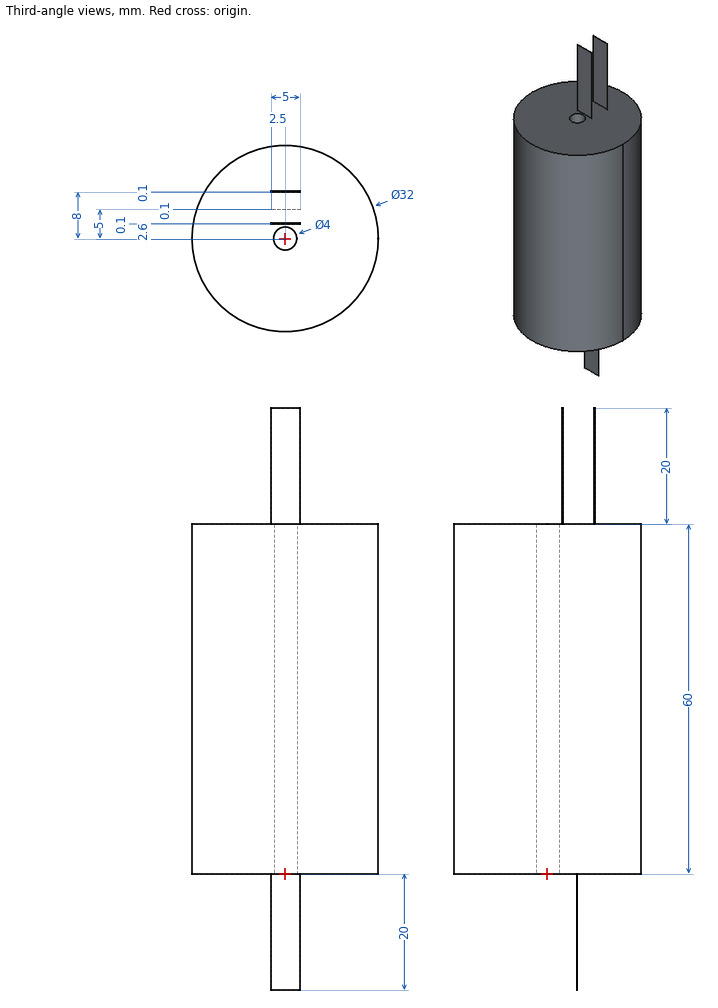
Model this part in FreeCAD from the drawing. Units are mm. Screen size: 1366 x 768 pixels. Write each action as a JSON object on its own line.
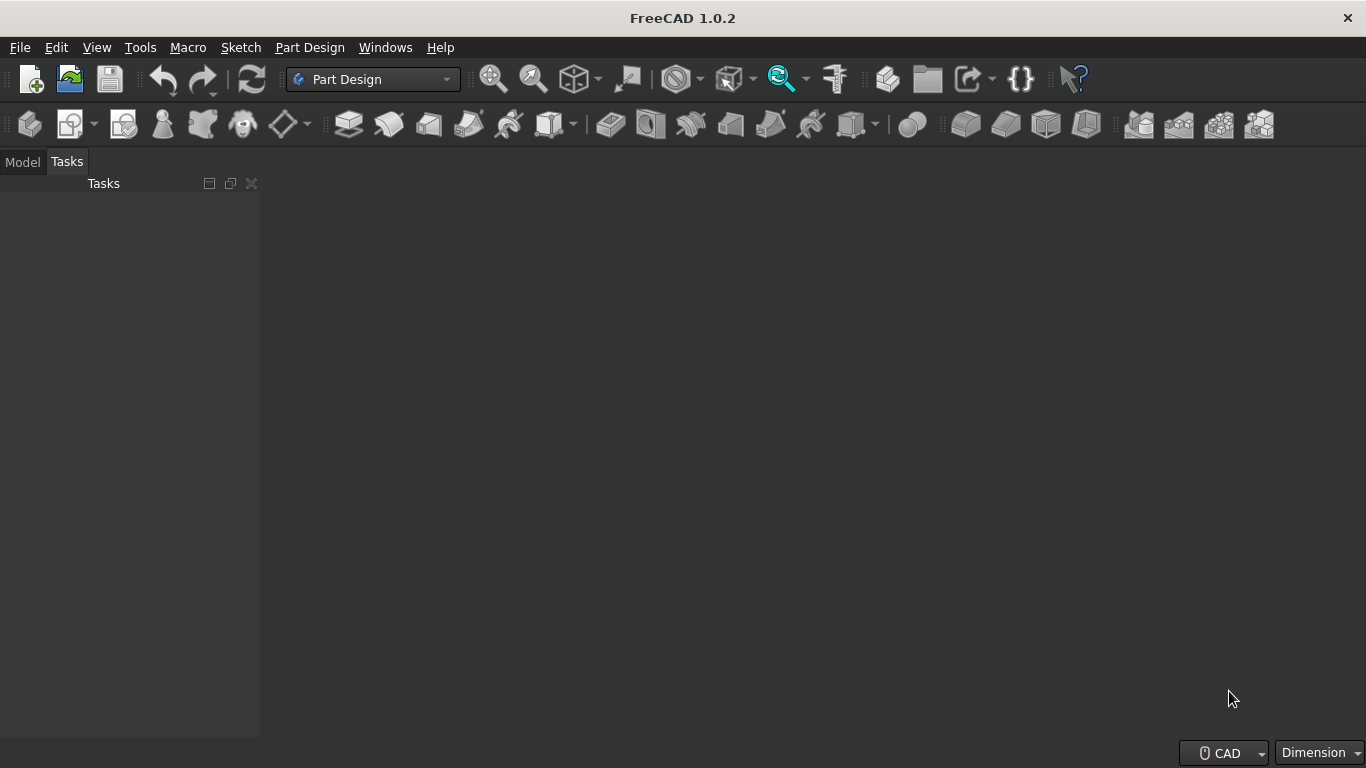
{"action": "left_click", "coordinate": [30, 80]}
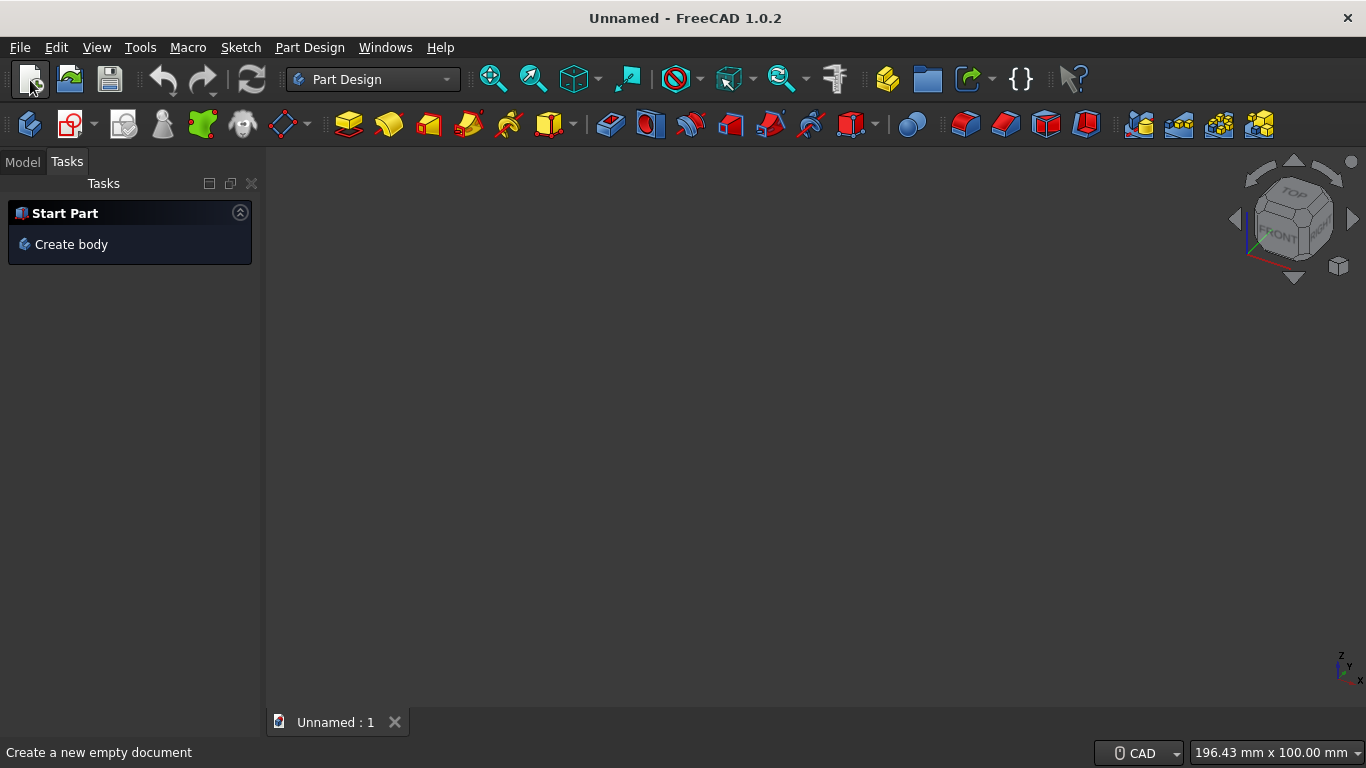
{"action": "left_click", "coordinate": [70, 124]}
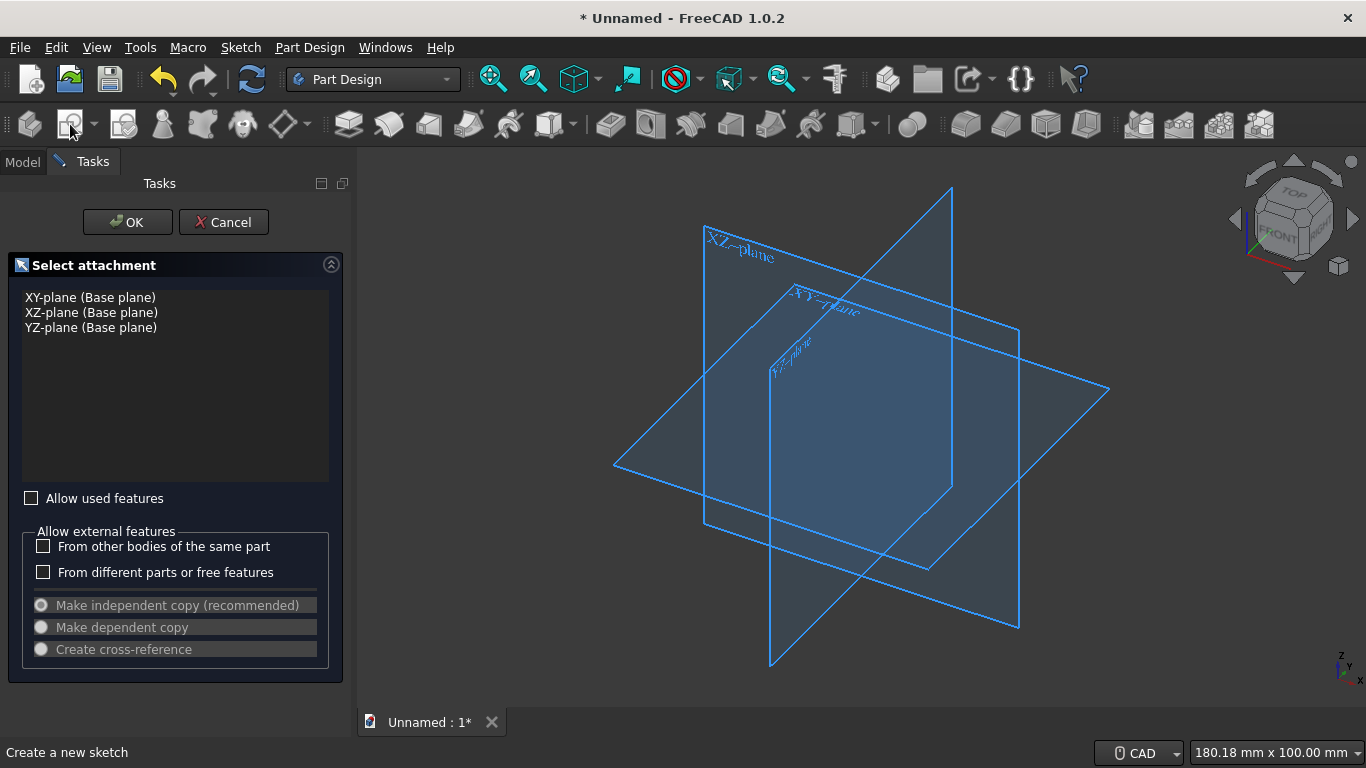
{"action": "left_click", "coordinate": [82, 298]}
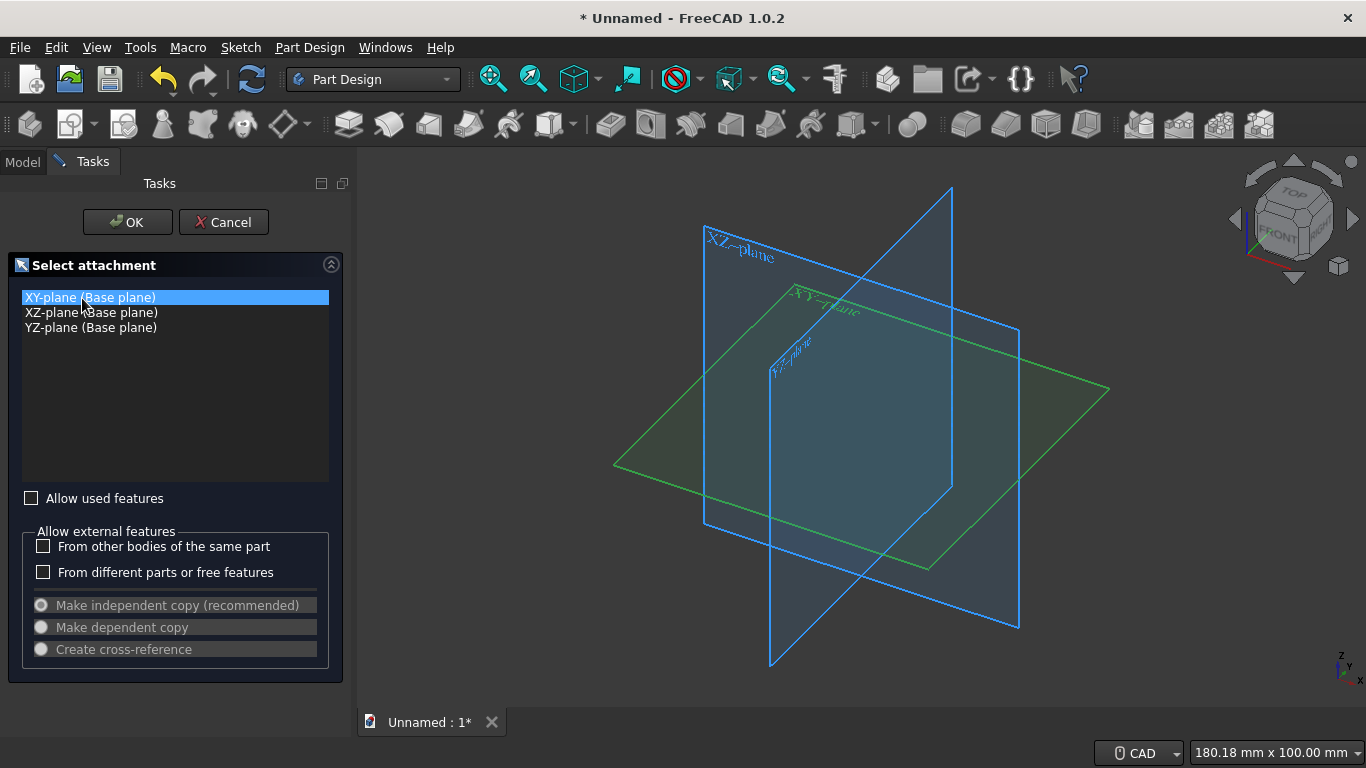
{"action": "left_click", "coordinate": [128, 222]}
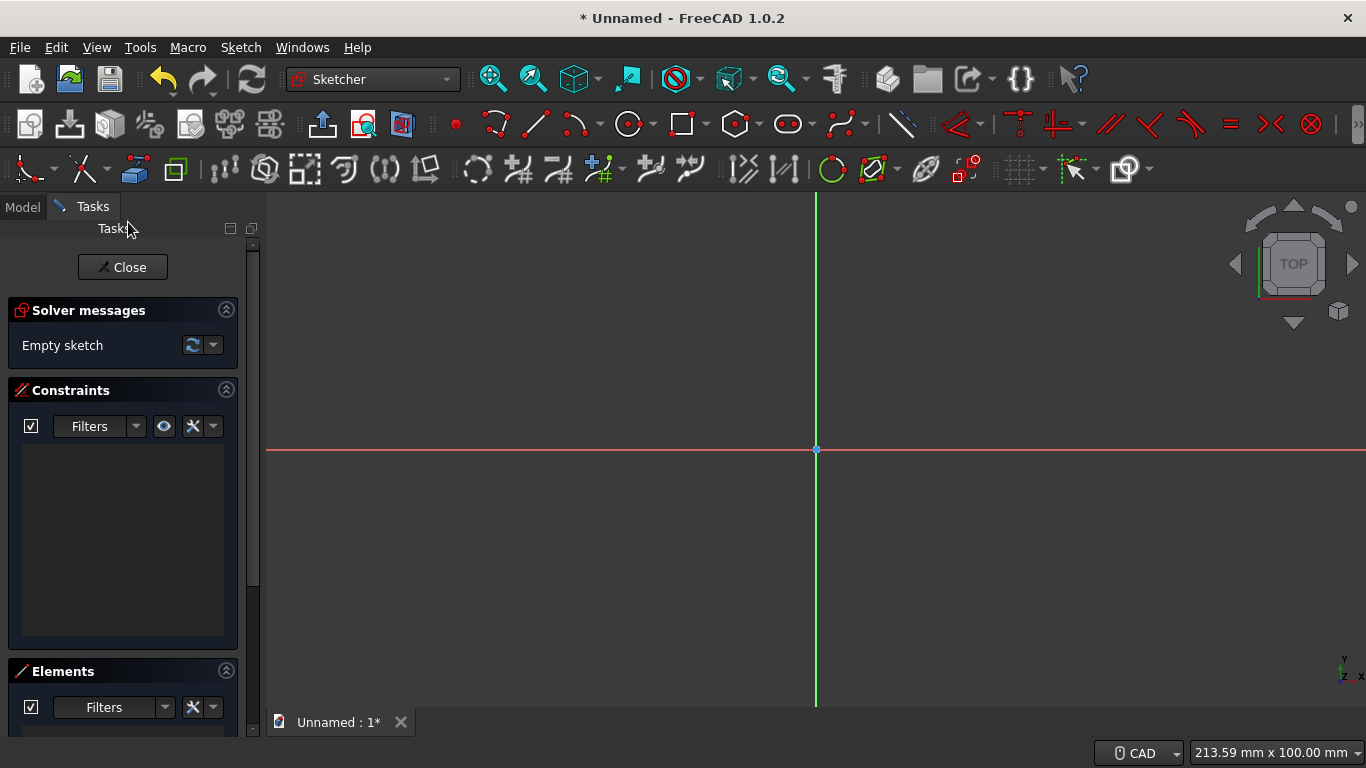
{"action": "scroll", "coordinate": [899, 449], "scroll_direction": "up", "scroll_amount": 3}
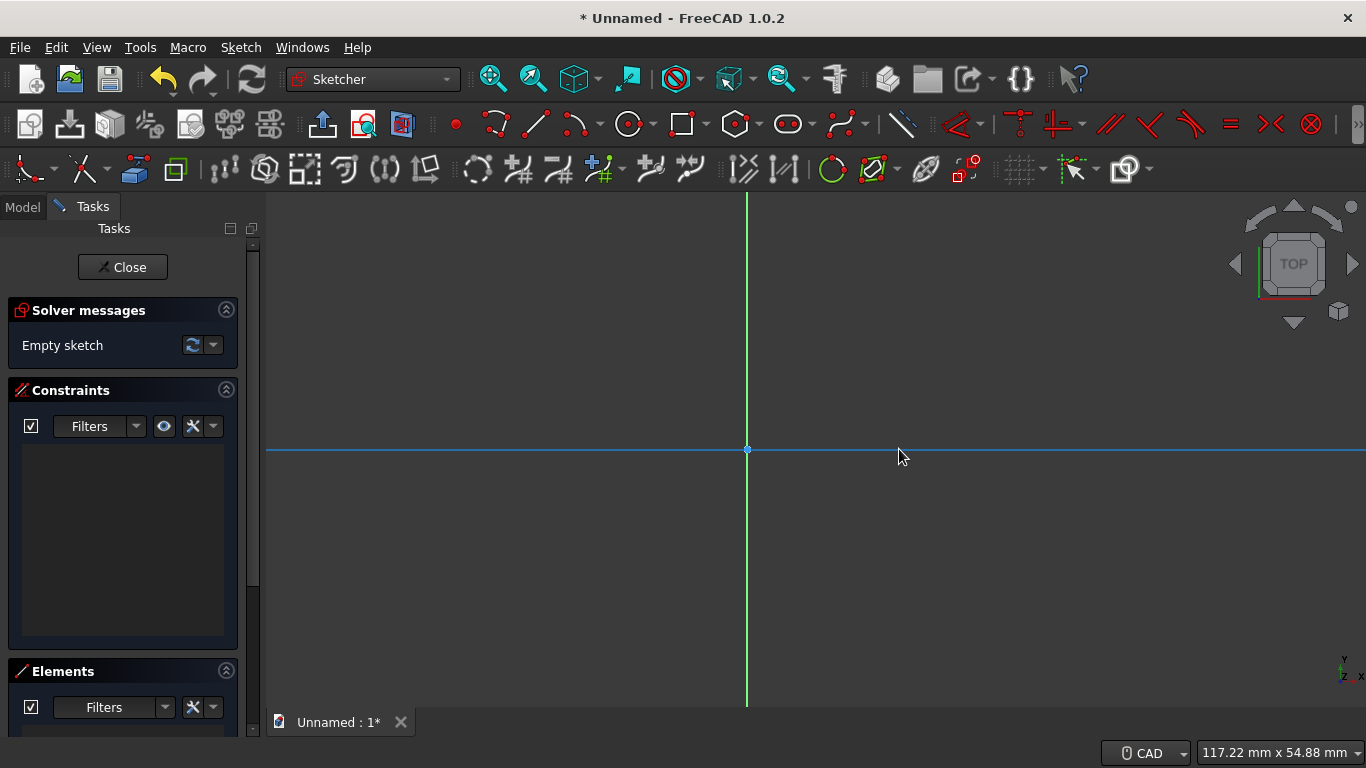
{"action": "left_click", "coordinate": [630, 124]}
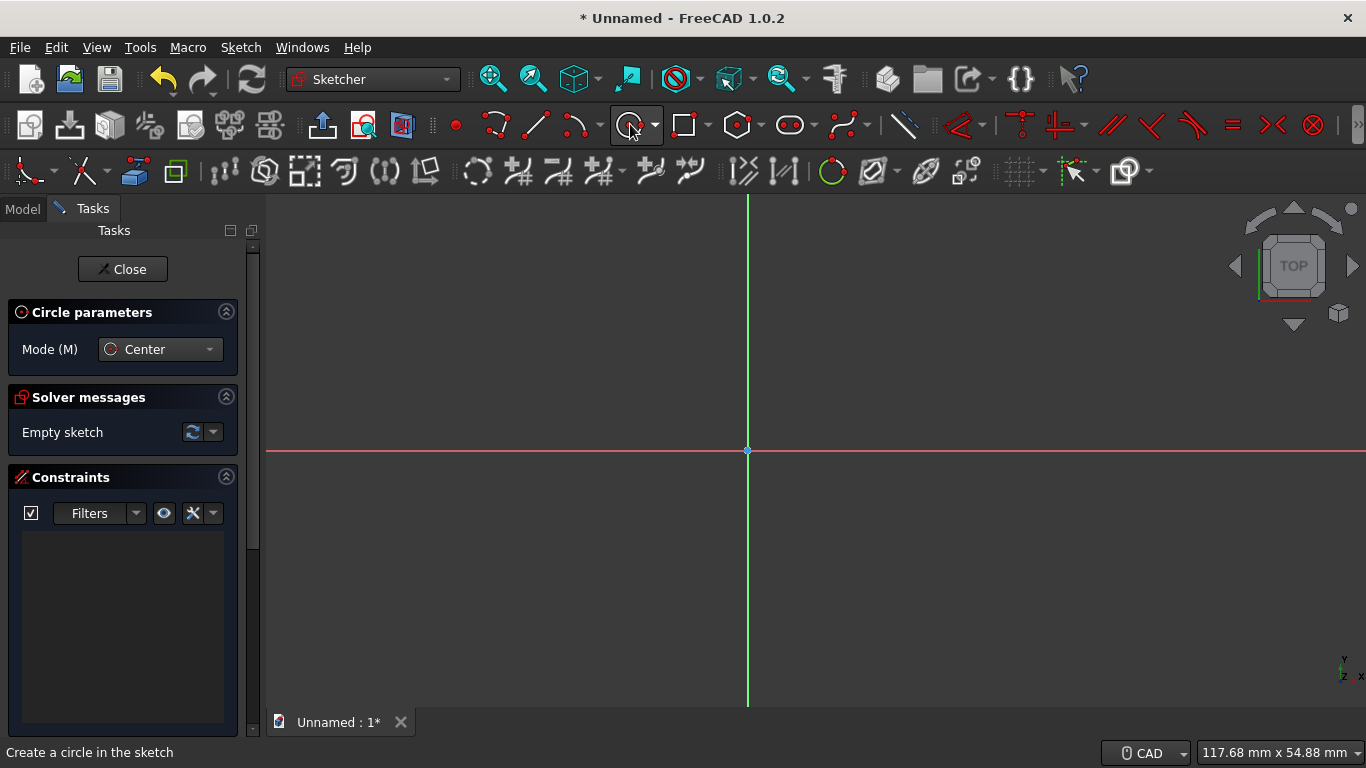
{"action": "left_click", "coordinate": [748, 450]}
{"action": "mouse_move", "coordinate": [853, 345]}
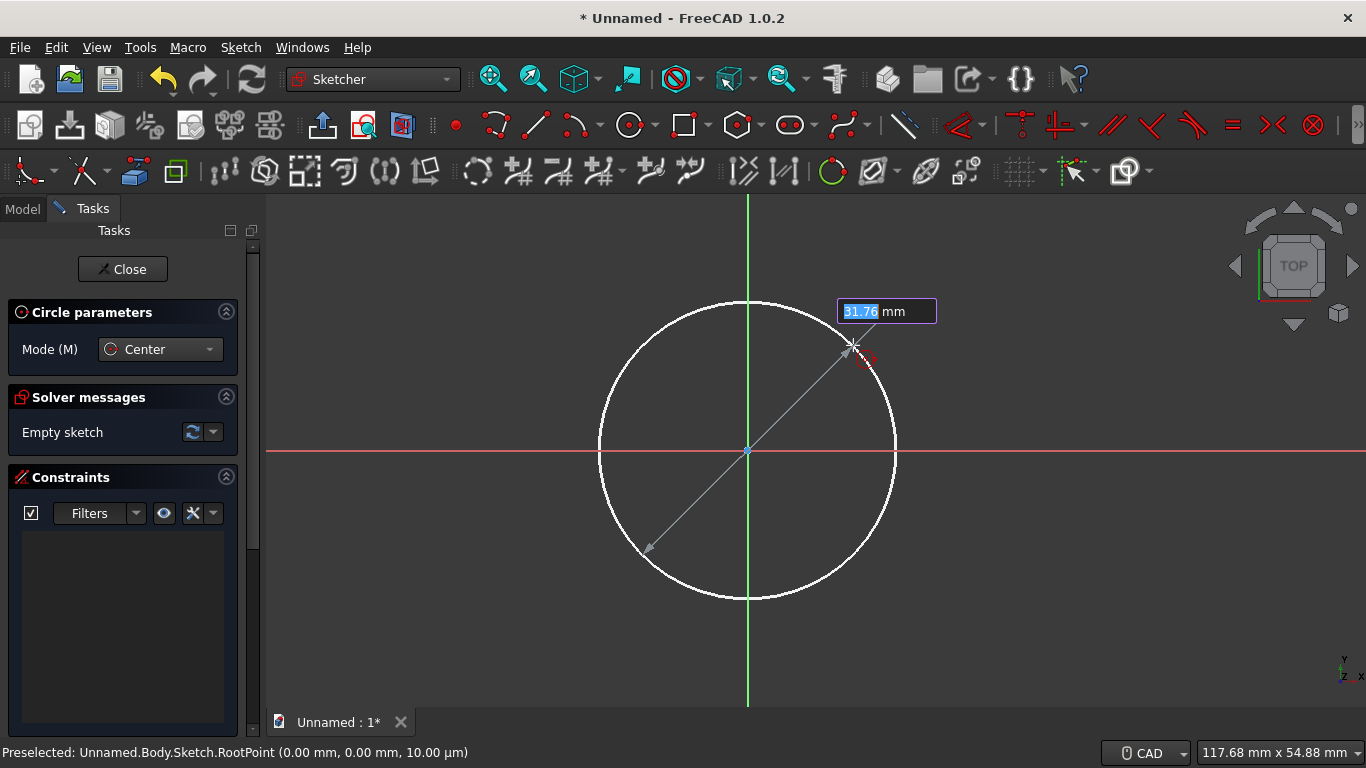
{"action": "type", "text": "32"}
{"action": "key", "text": "Return"}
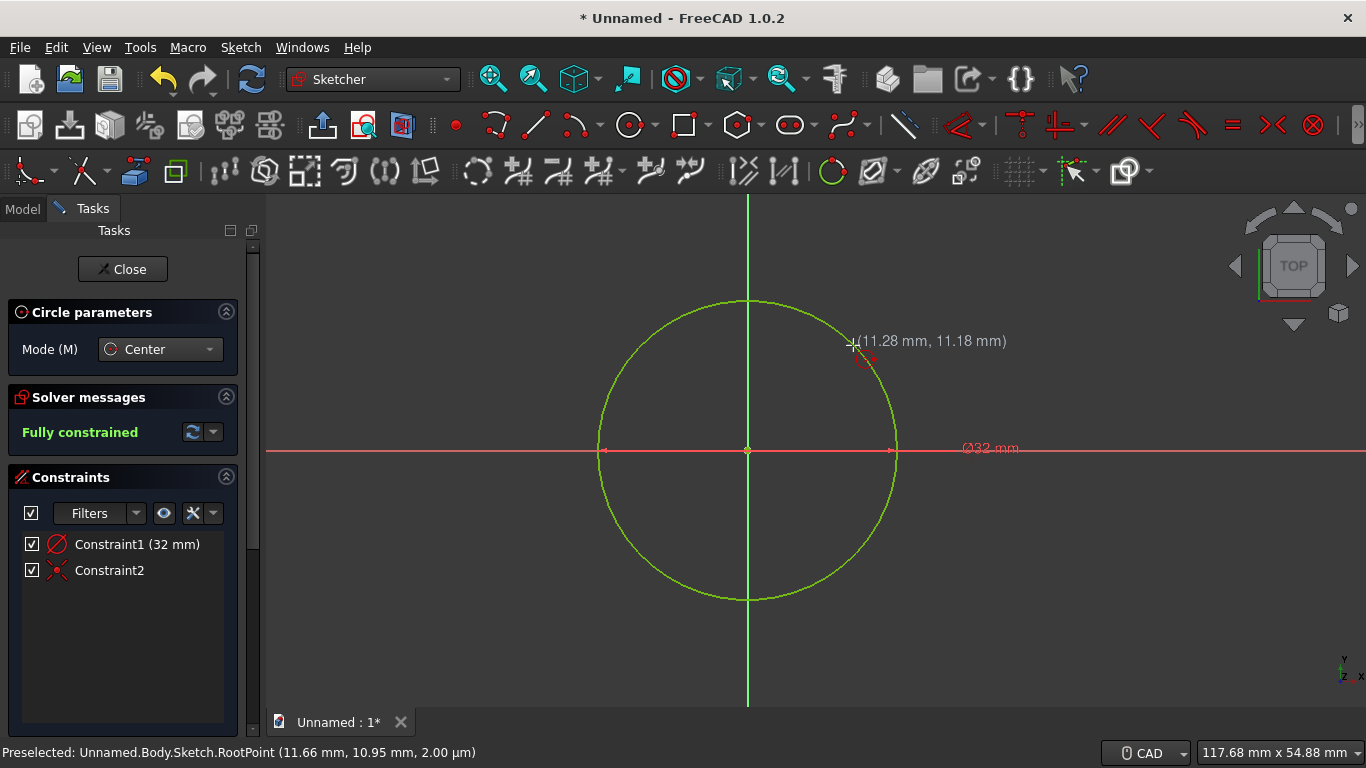
{"action": "left_click", "coordinate": [748, 450]}
{"action": "mouse_move", "coordinate": [761, 437]}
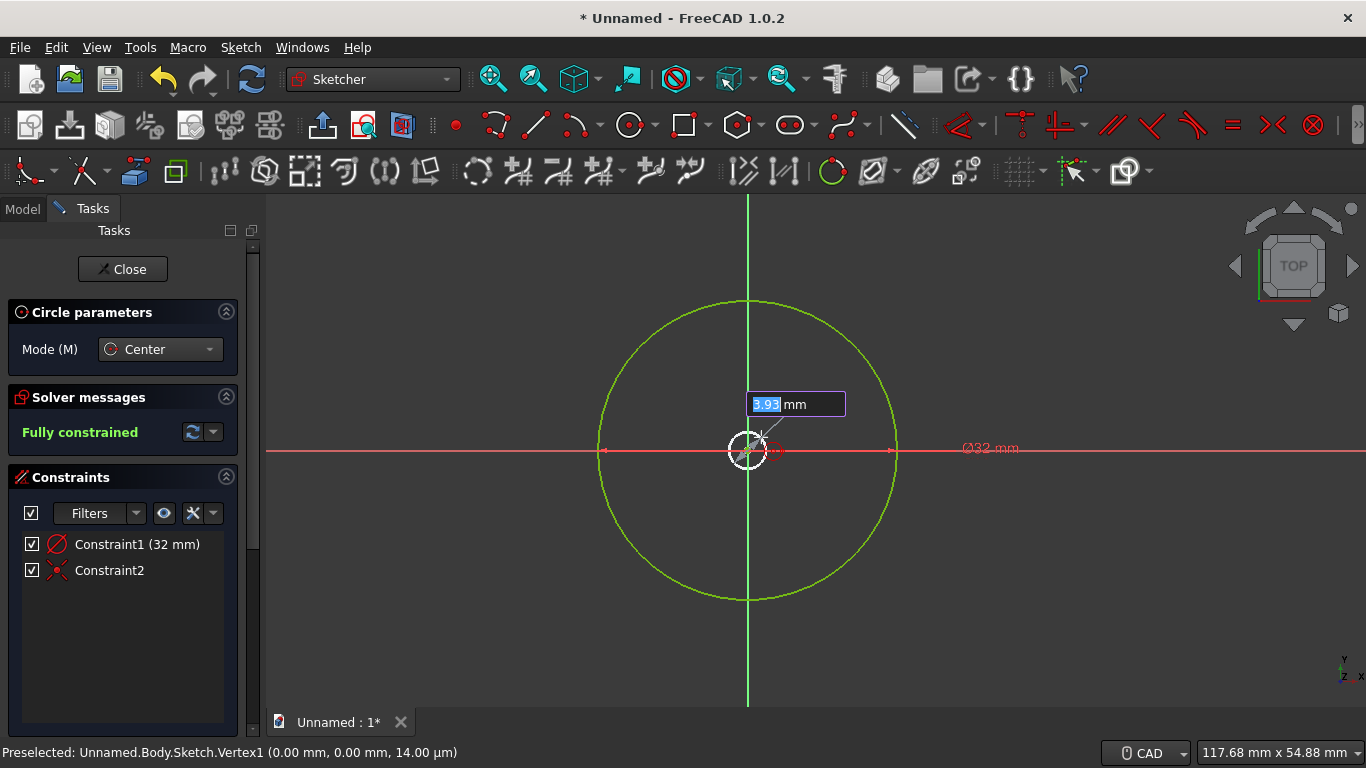
{"action": "type", "text": "4"}
{"action": "key", "text": "Return"}
{"action": "key", "text": "Escape"}